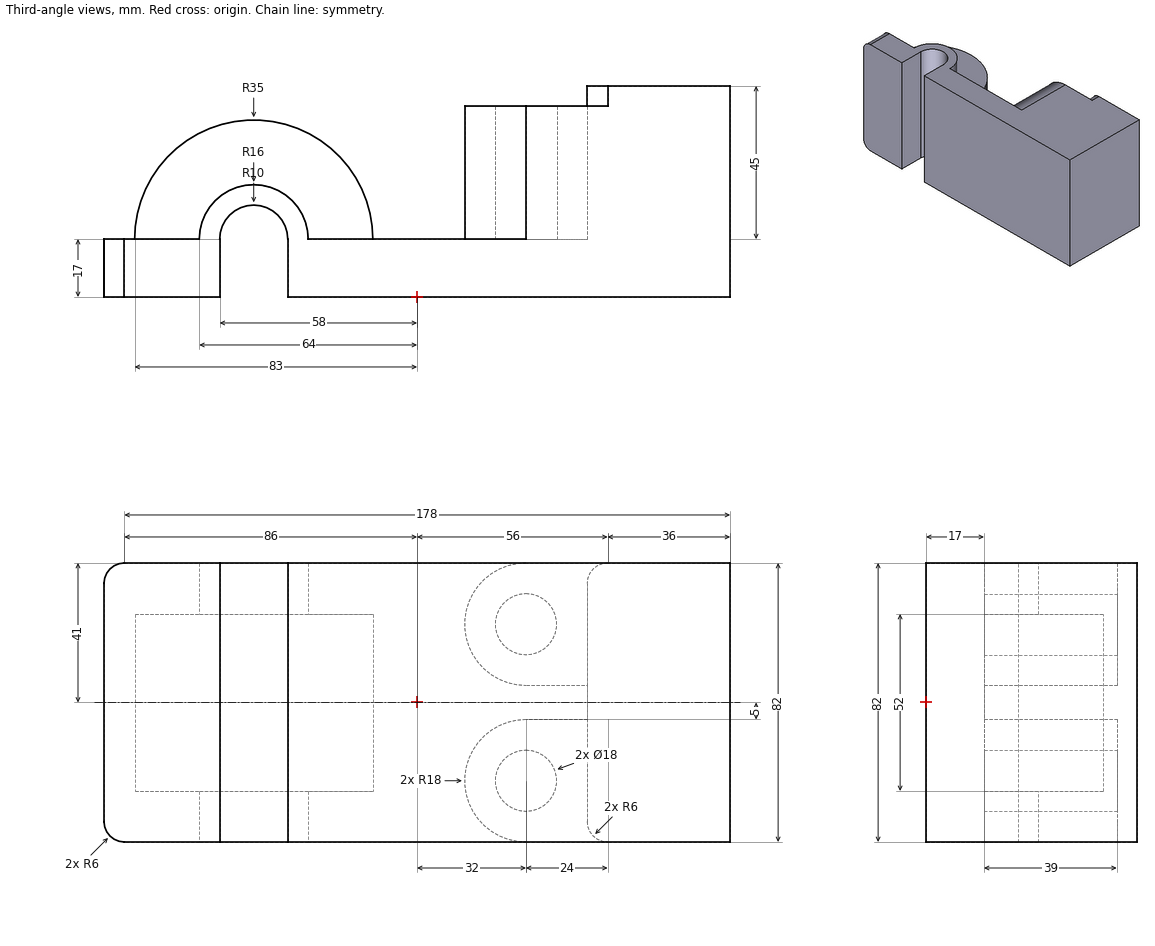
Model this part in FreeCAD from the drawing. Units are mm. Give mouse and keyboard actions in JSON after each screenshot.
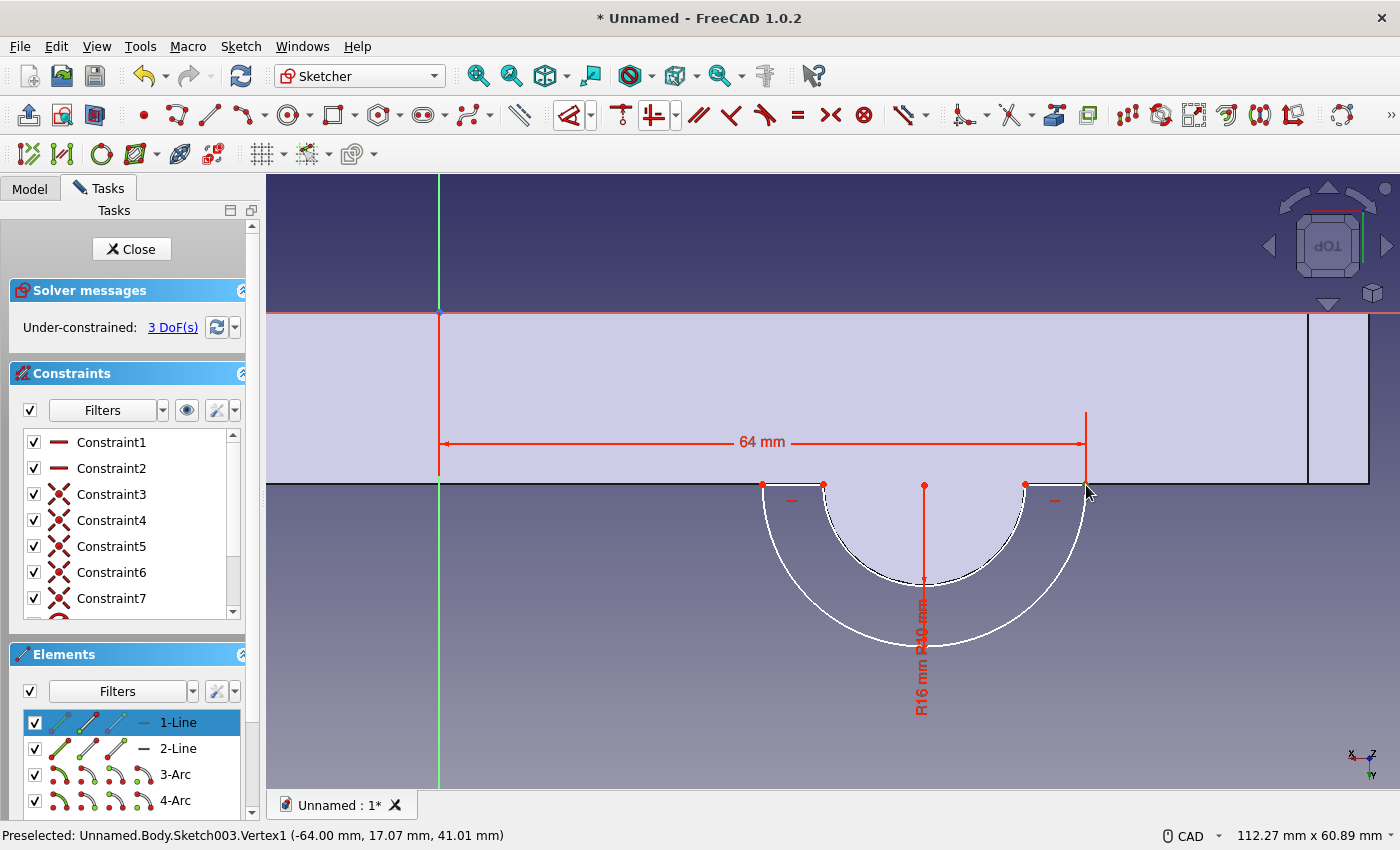
{"action": "key", "text": "i"}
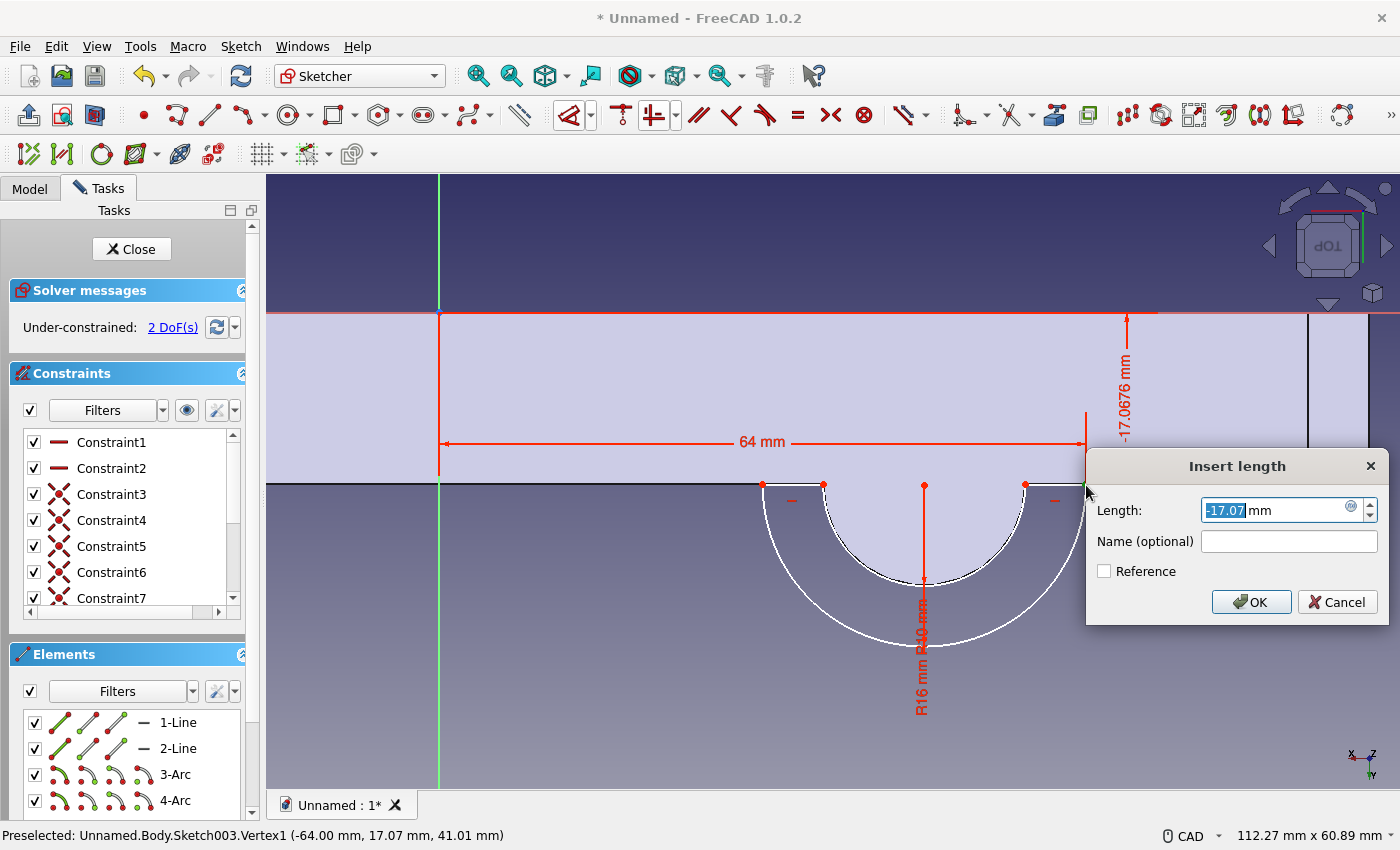
{"action": "type", "text": "-17"}
{"action": "key", "text": "Return"}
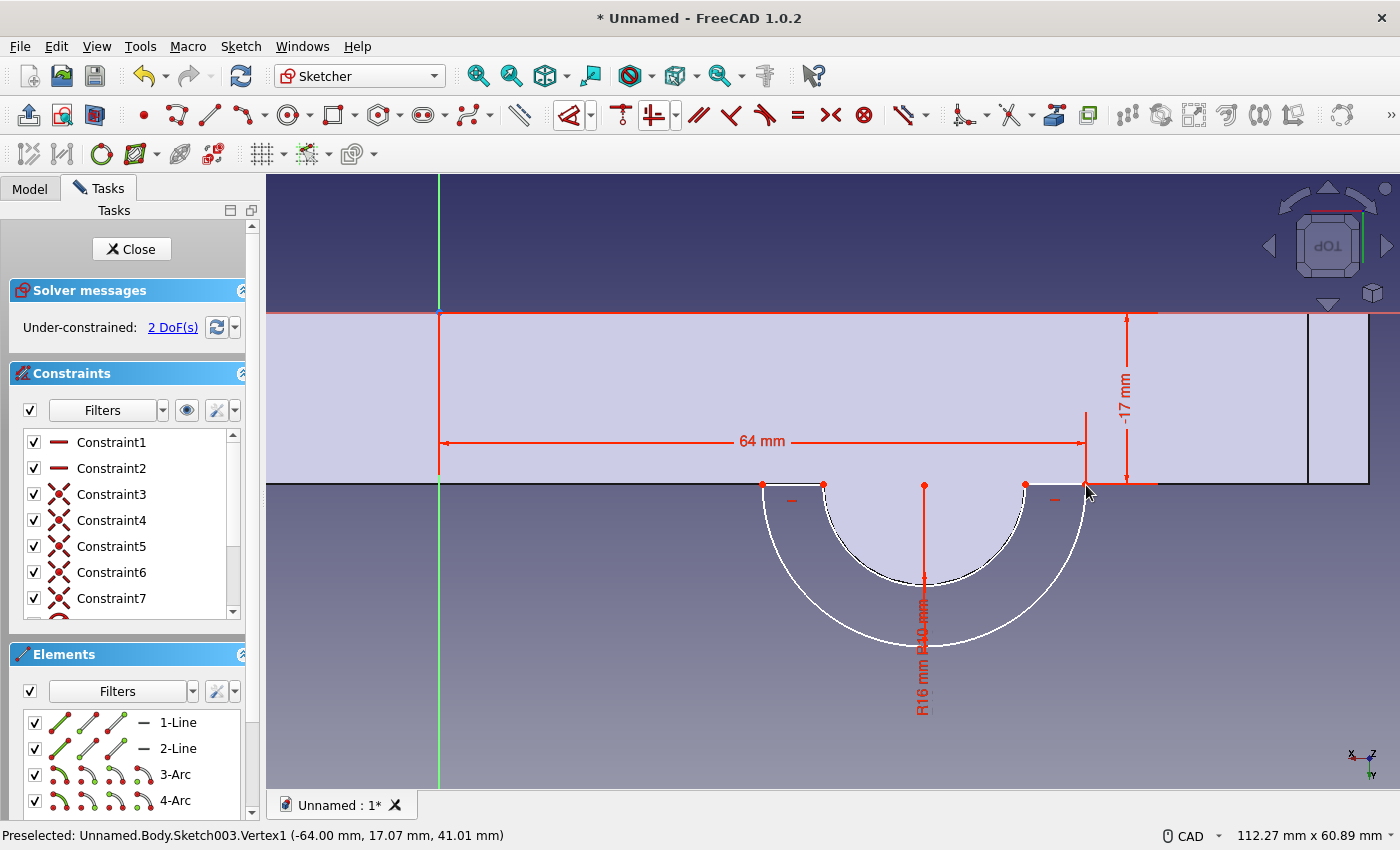
{"action": "left_click", "coordinate": [823, 485]}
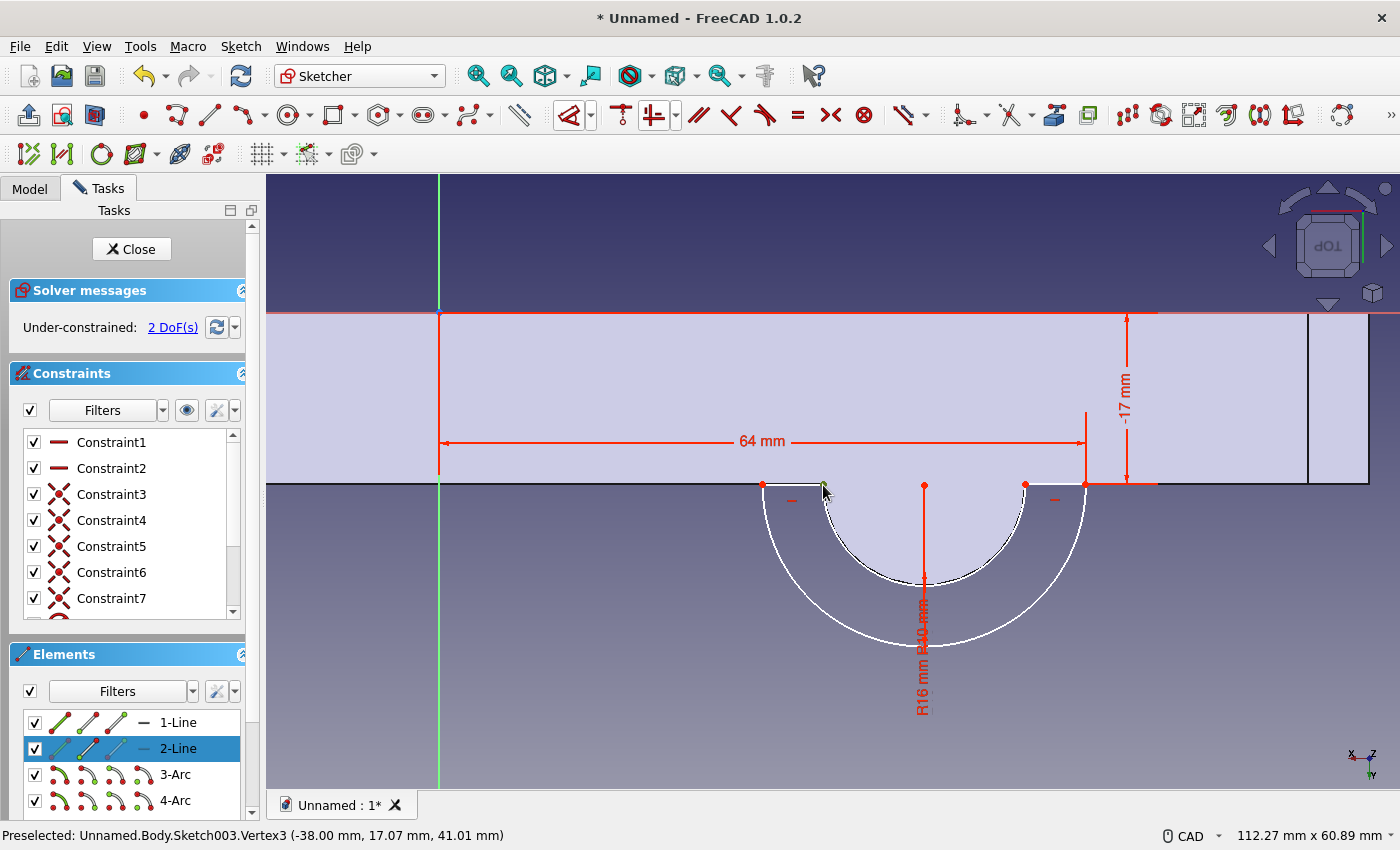
{"action": "key", "text": "i"}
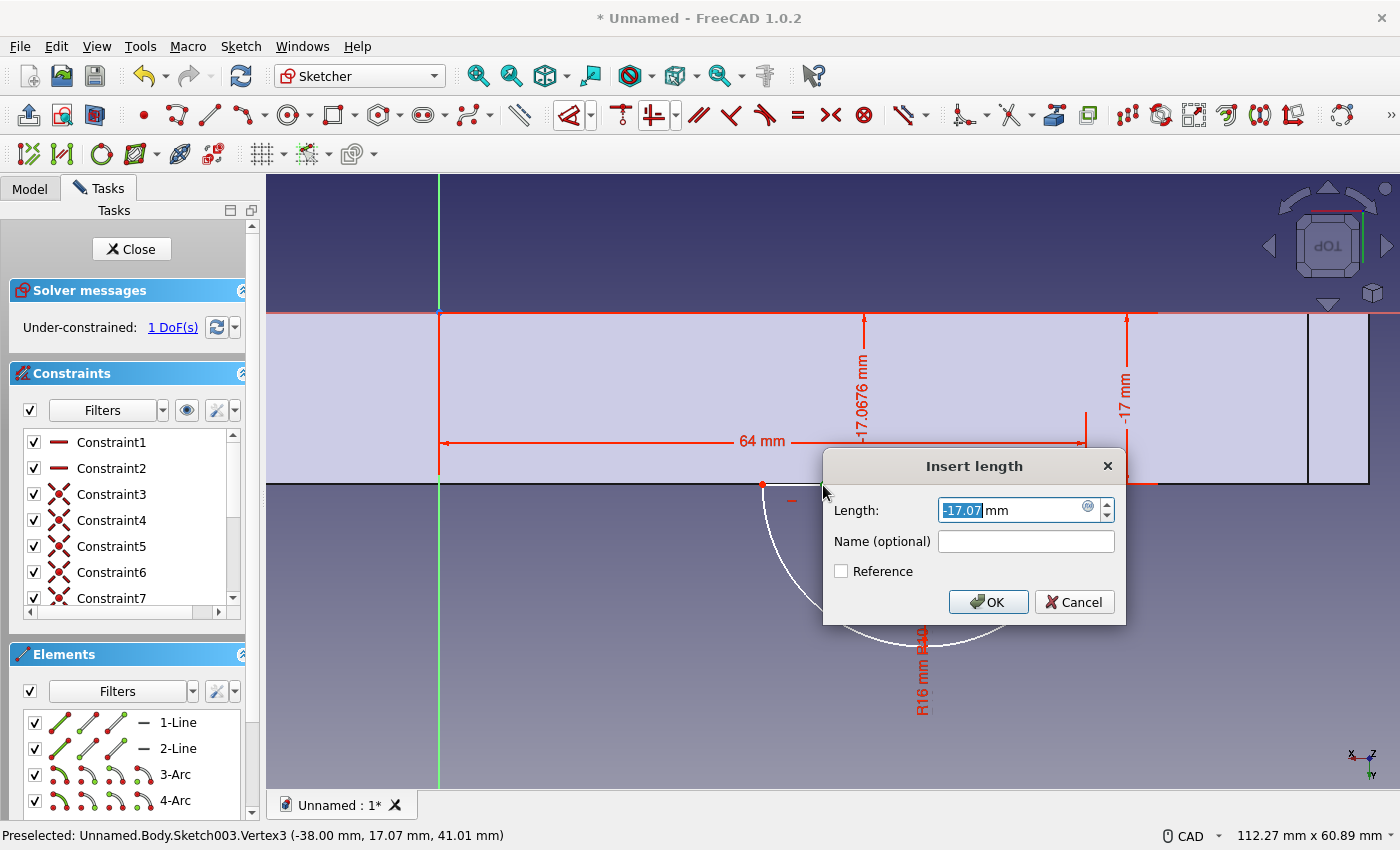
{"action": "type", "text": "-17"}
{"action": "key", "text": "Return"}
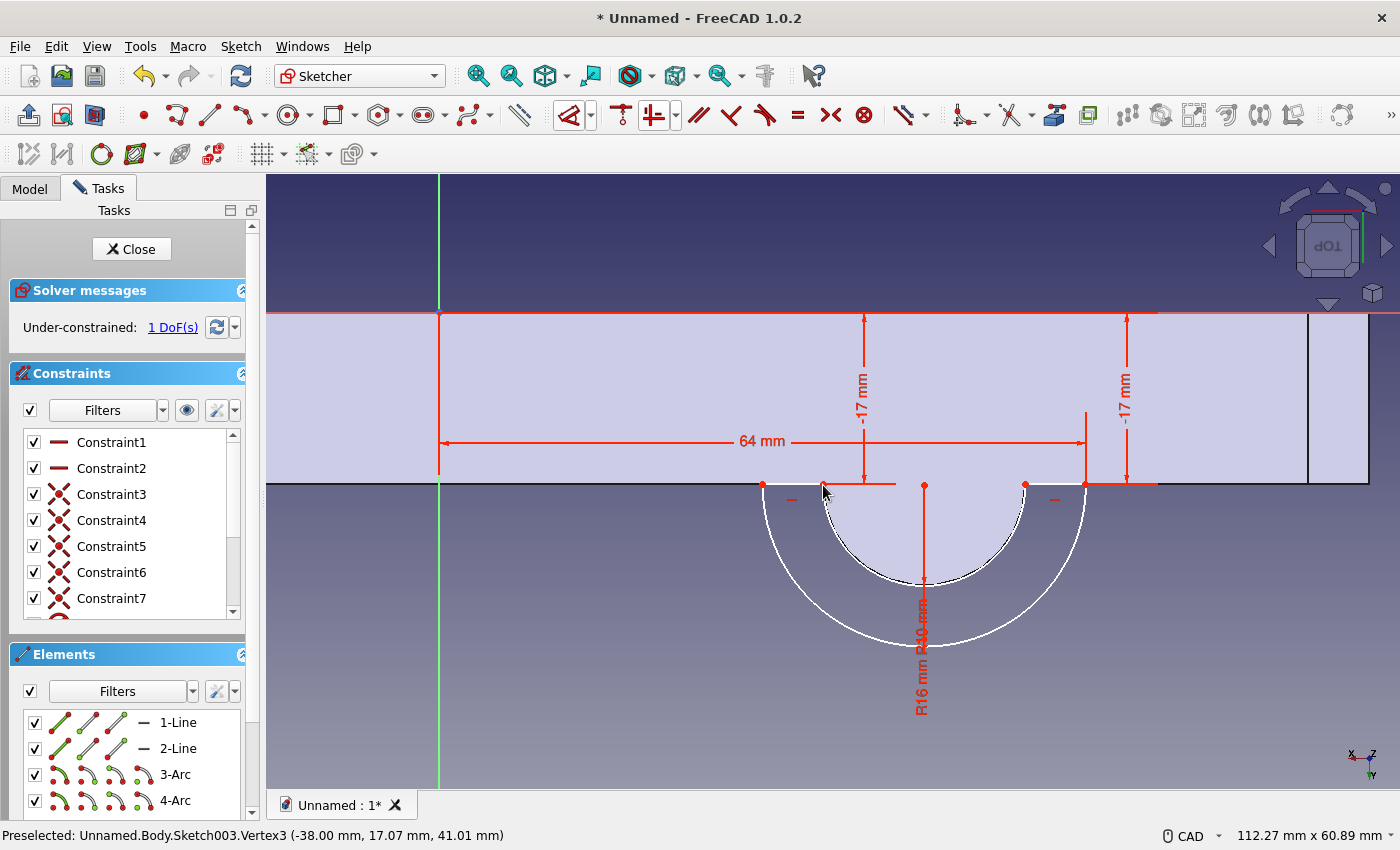
{"action": "left_click", "coordinate": [924, 485]}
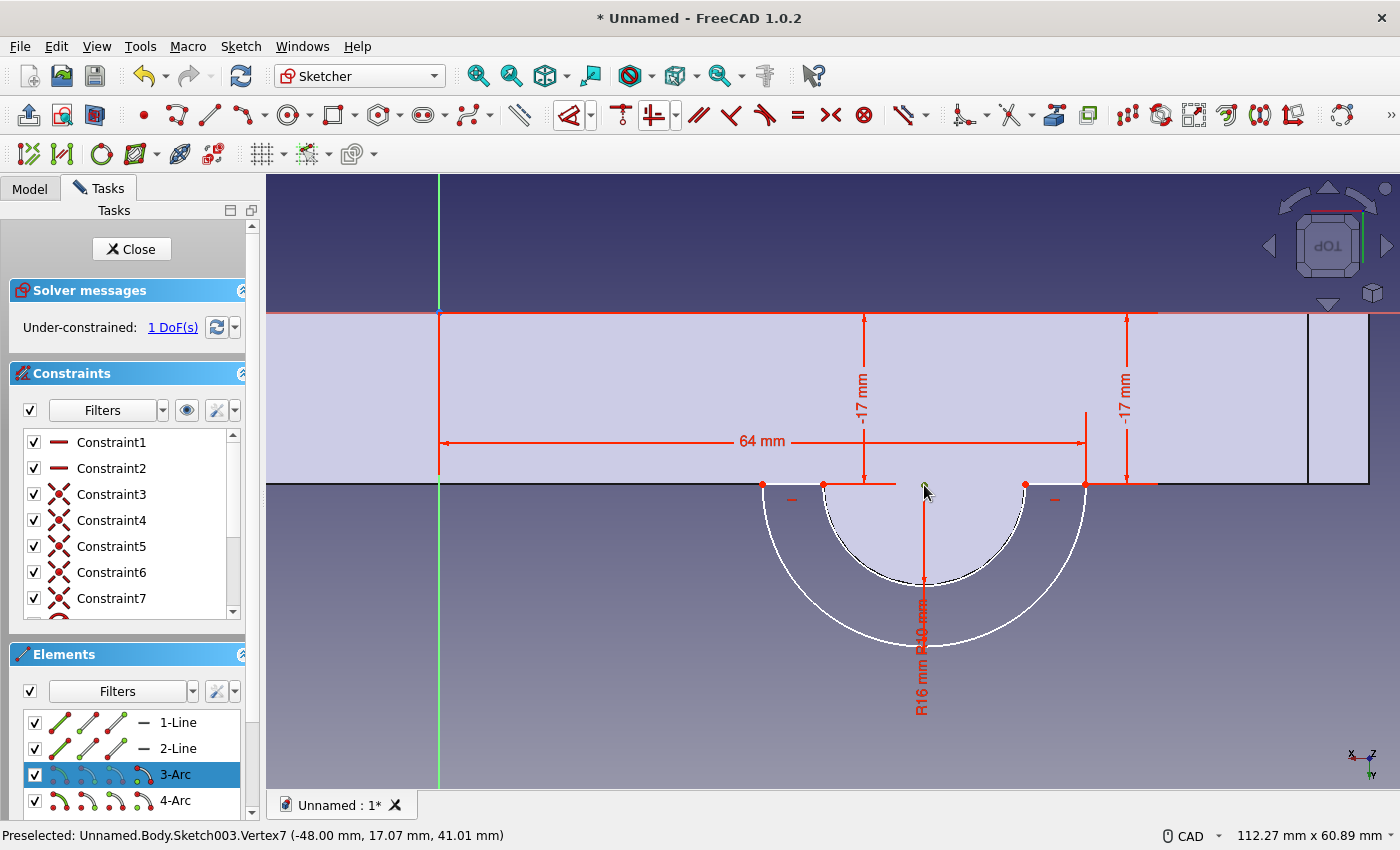
{"action": "left_click", "coordinate": [590, 116]}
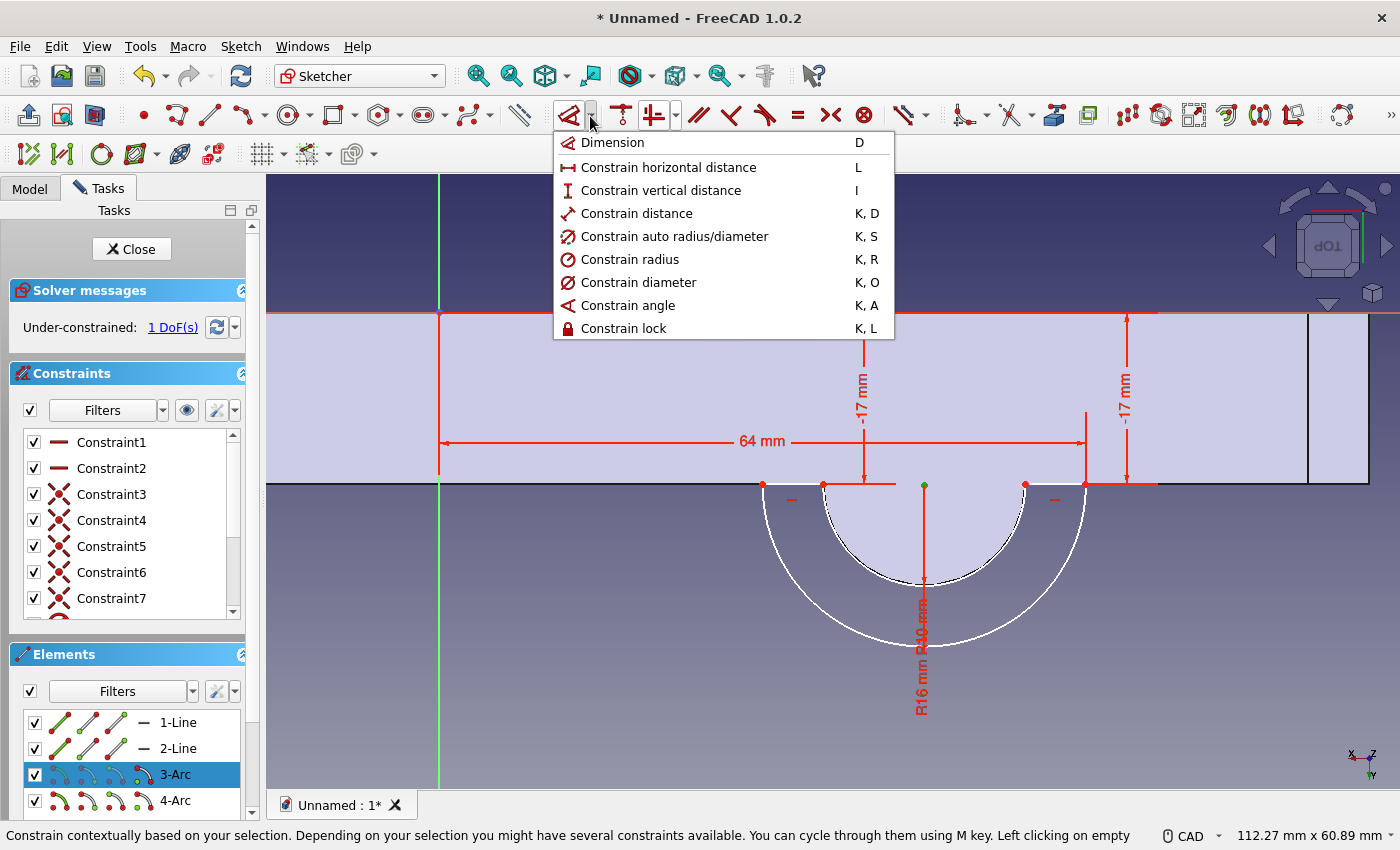
{"action": "left_click", "coordinate": [724, 190]}